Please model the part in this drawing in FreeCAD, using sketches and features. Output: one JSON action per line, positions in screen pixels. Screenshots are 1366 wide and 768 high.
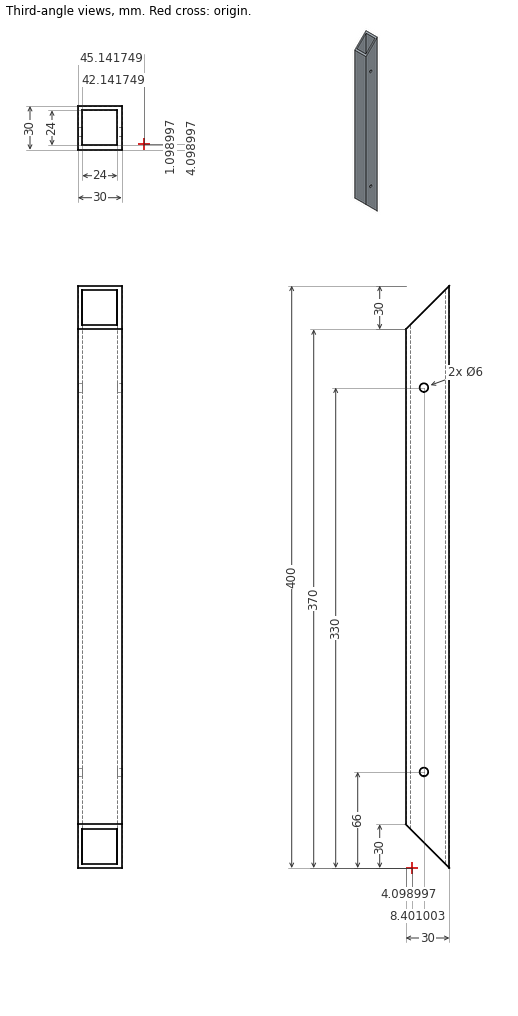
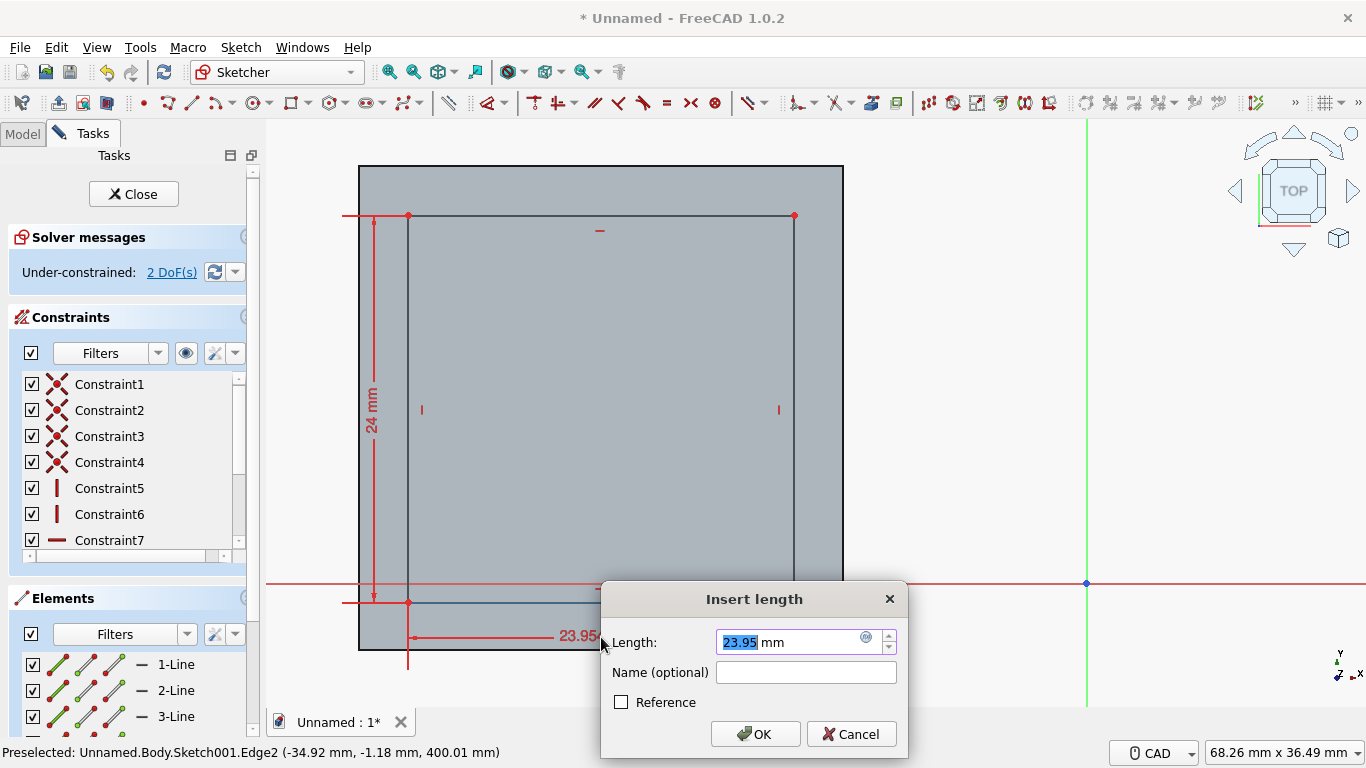
{"action": "type", "text": "24"}
{"action": "key", "text": "Return"}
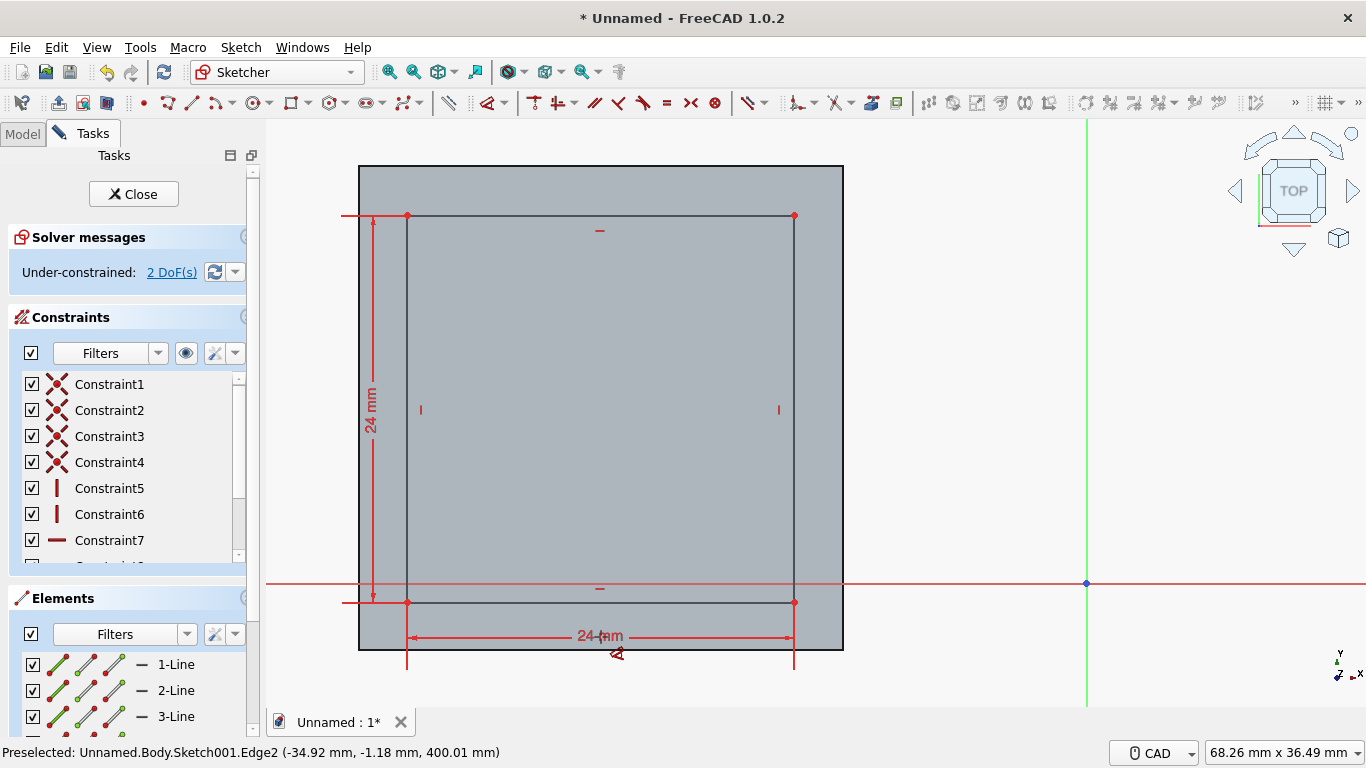
{"action": "scroll", "coordinate": [407, 603], "scroll_direction": "up", "scroll_amount": 5}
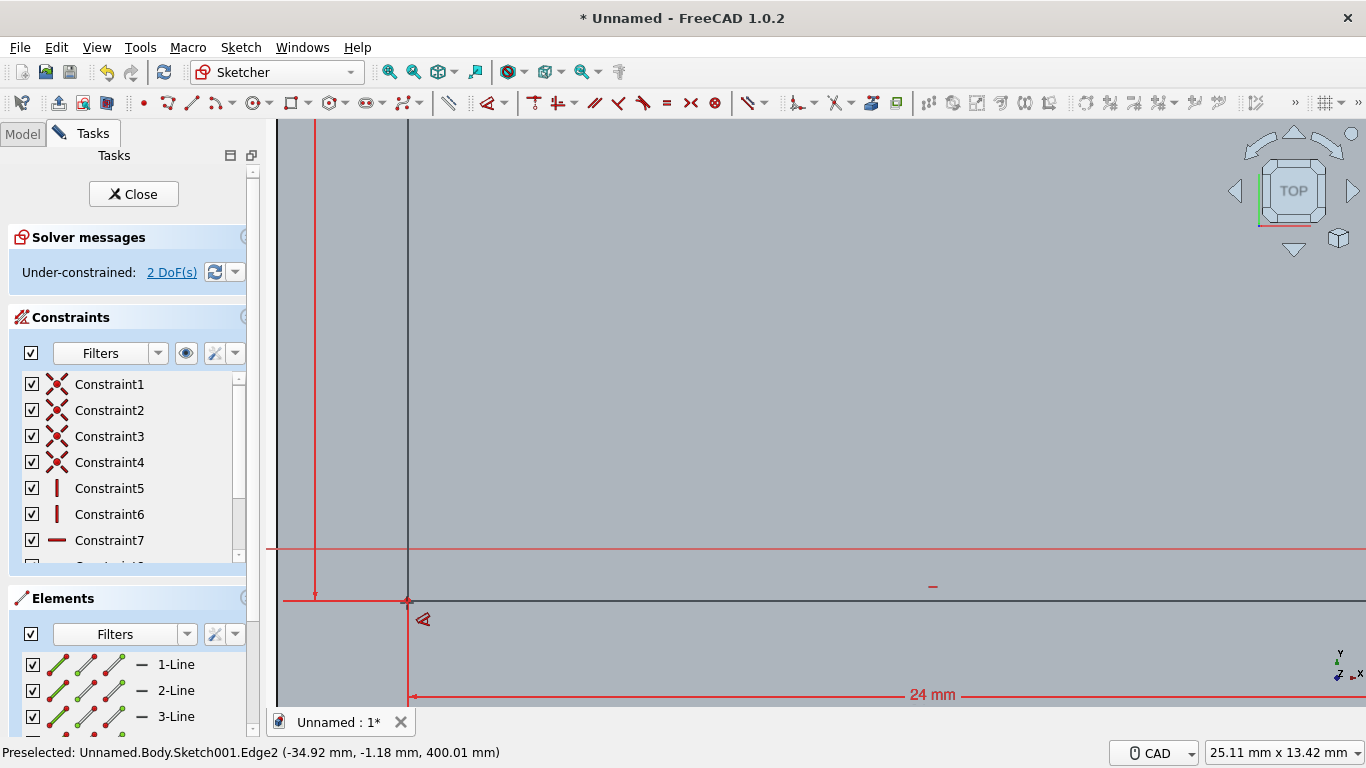
{"action": "left_click", "coordinate": [408, 601]}
{"action": "left_click", "coordinate": [374, 575]}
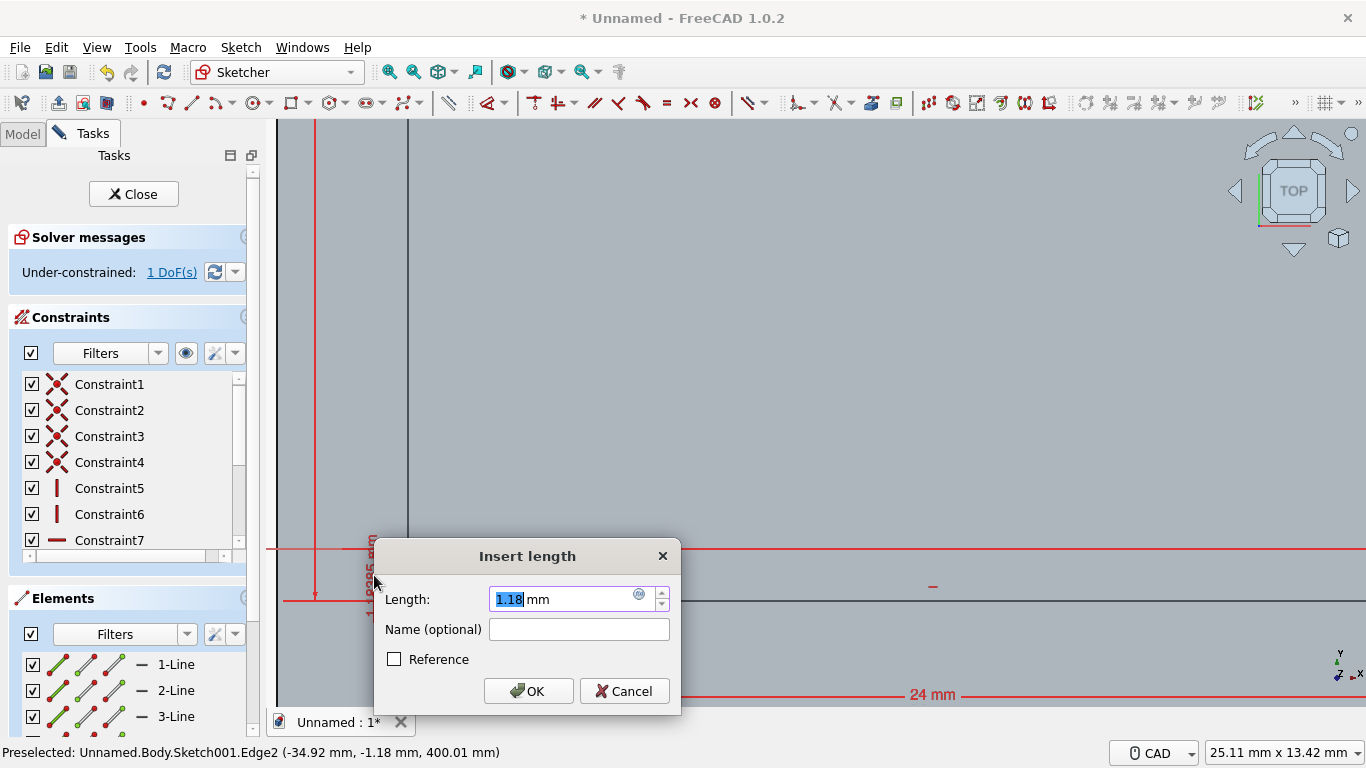
{"action": "type", "text": "1.098997"}
{"action": "key", "text": "Return"}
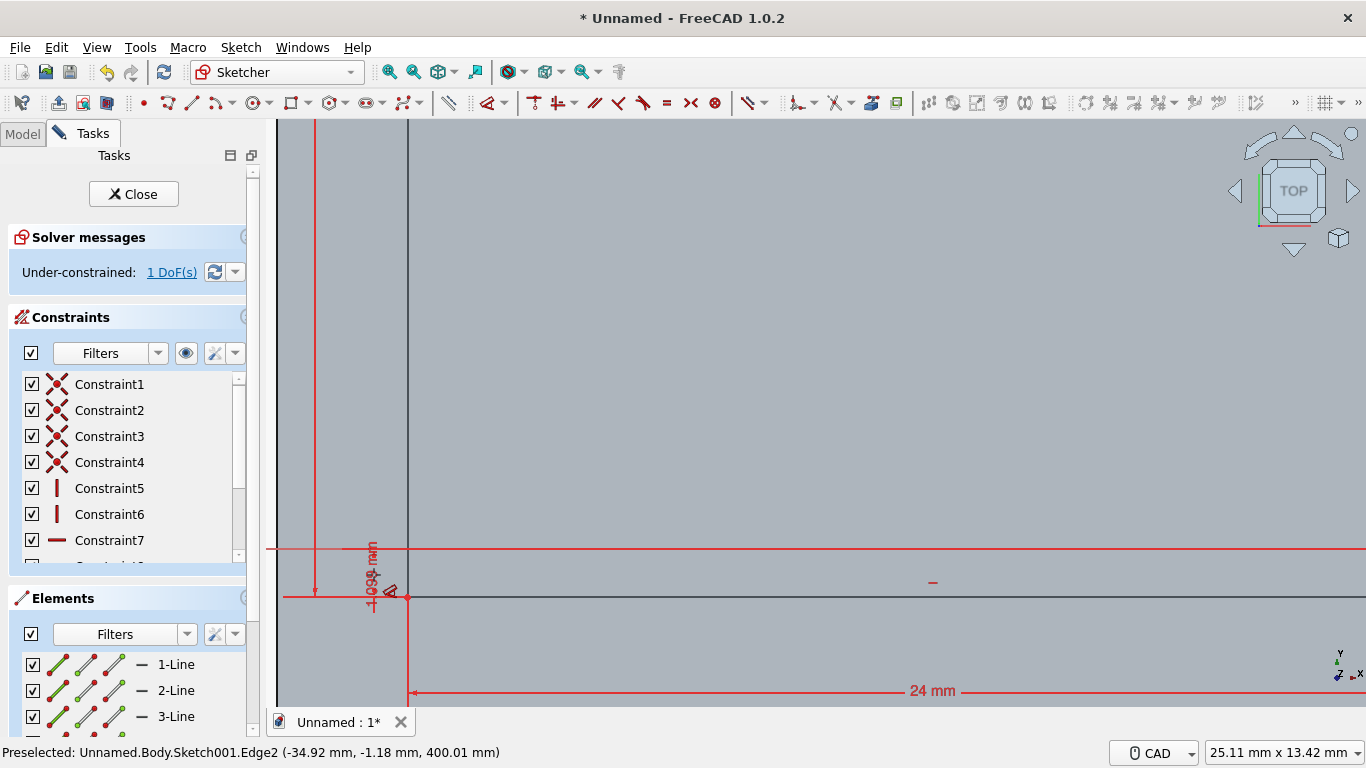
{"action": "scroll", "coordinate": [408, 612], "scroll_direction": "down", "scroll_amount": 5}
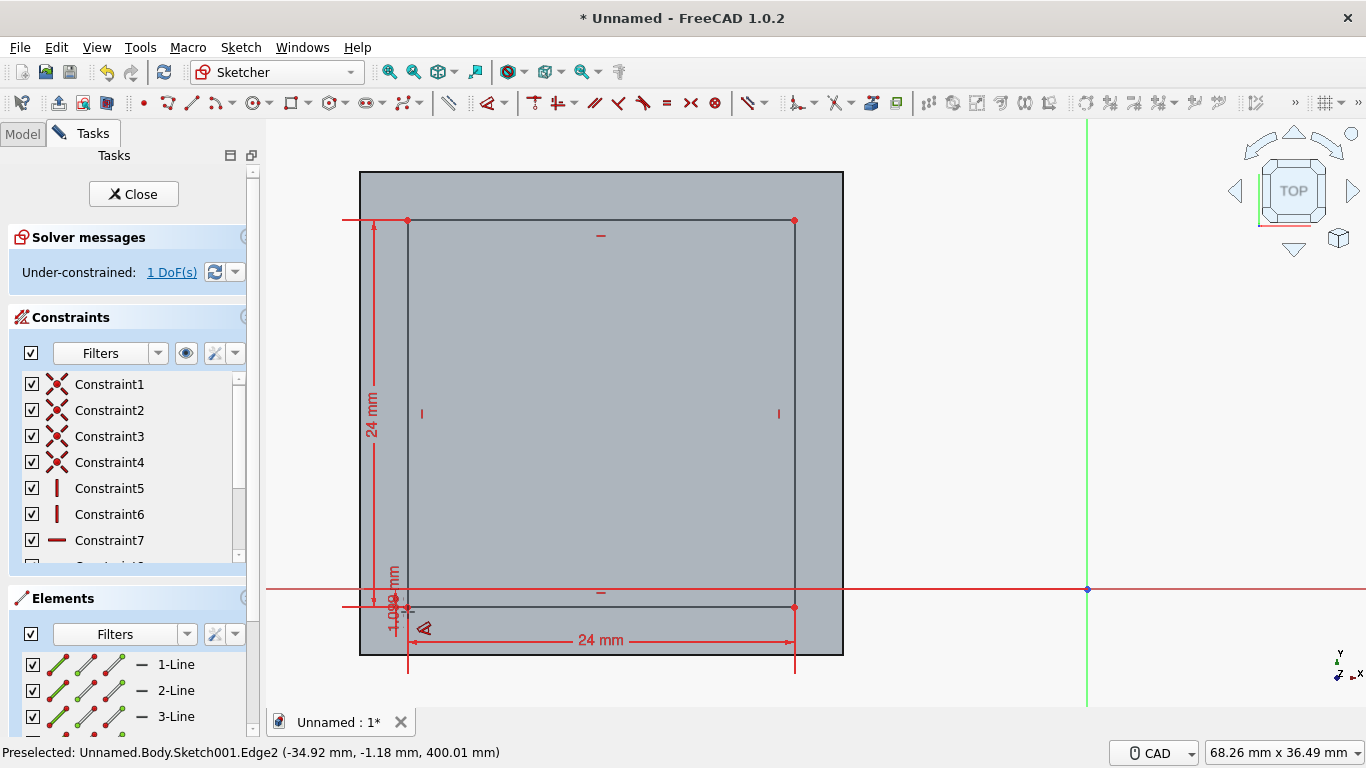
{"action": "left_click", "coordinate": [408, 220]}
{"action": "left_click", "coordinate": [748, 186]}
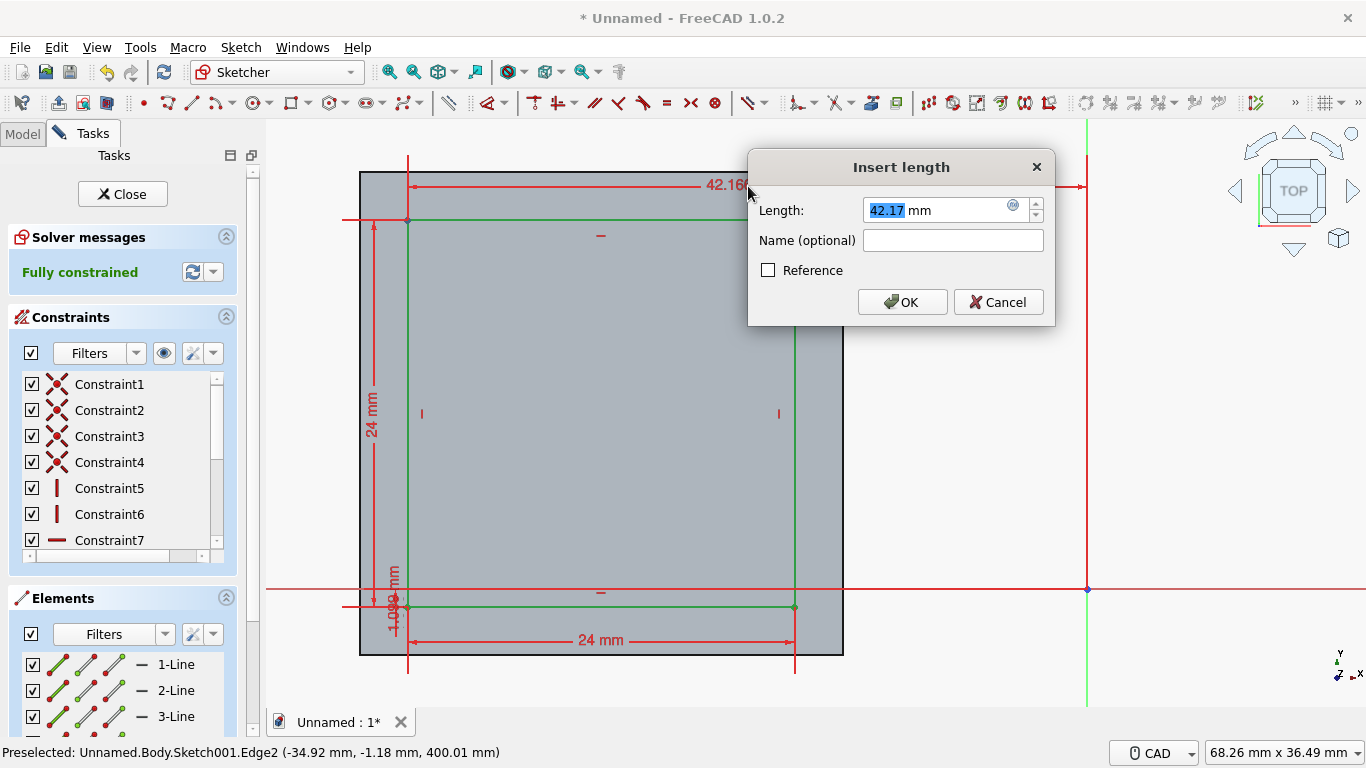
{"action": "type", "text": "42.141749"}
{"action": "key", "text": "Return"}
{"action": "key", "text": "Escape"}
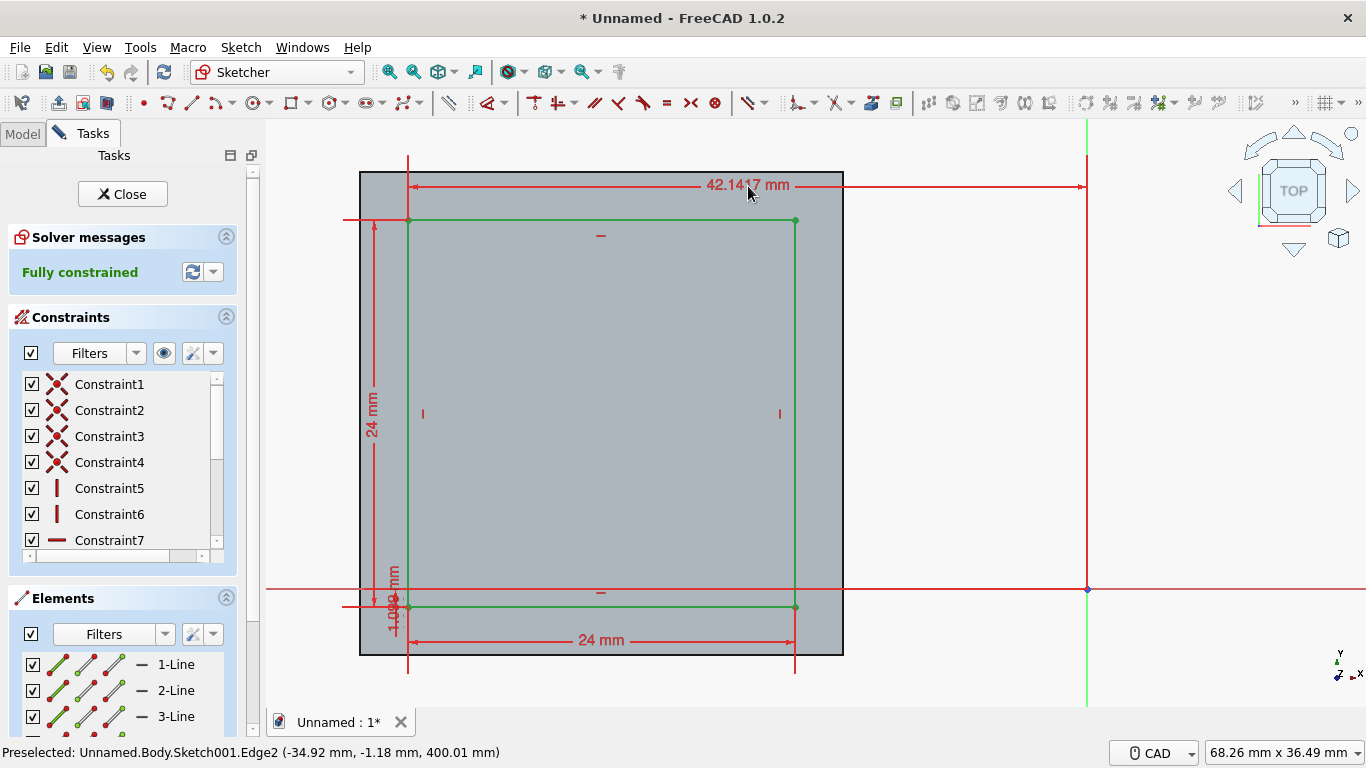
{"action": "left_click", "coordinate": [123, 194]}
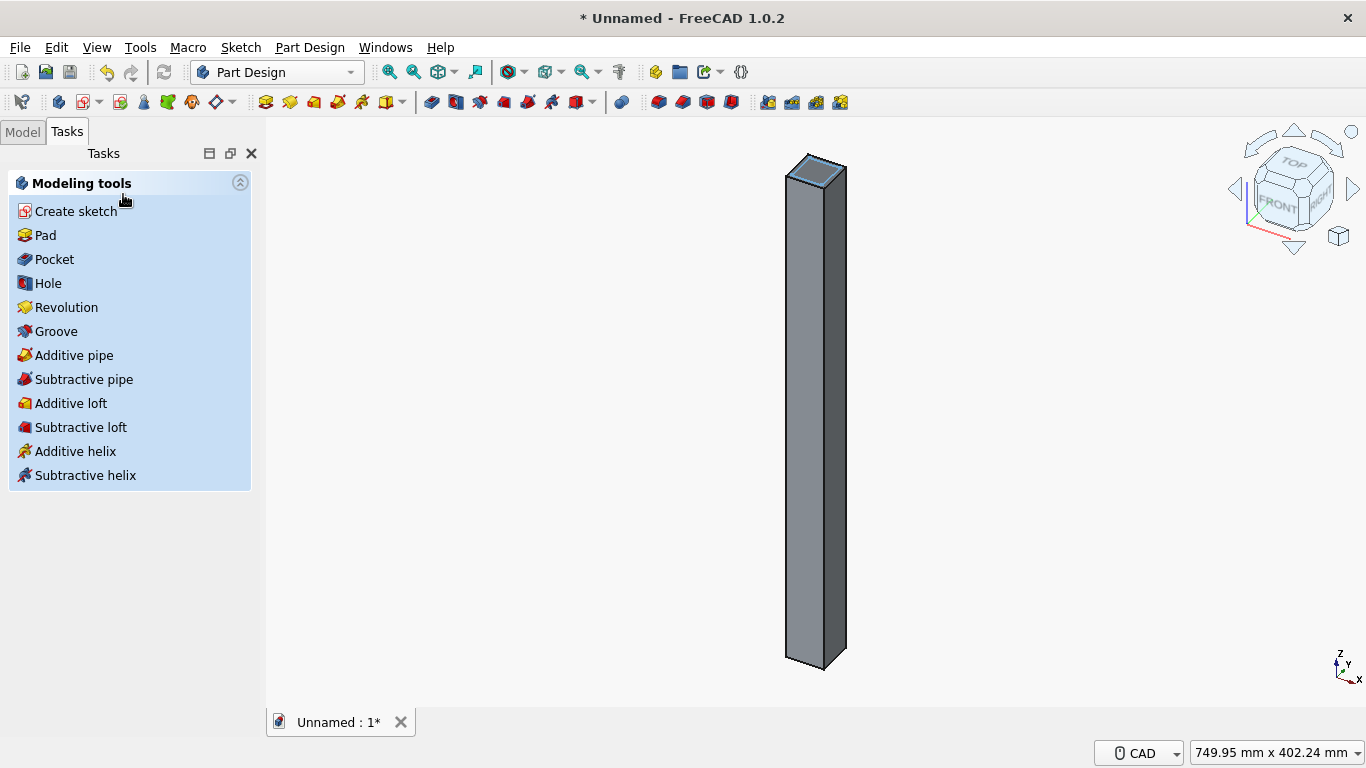
{"action": "left_click", "coordinate": [432, 102]}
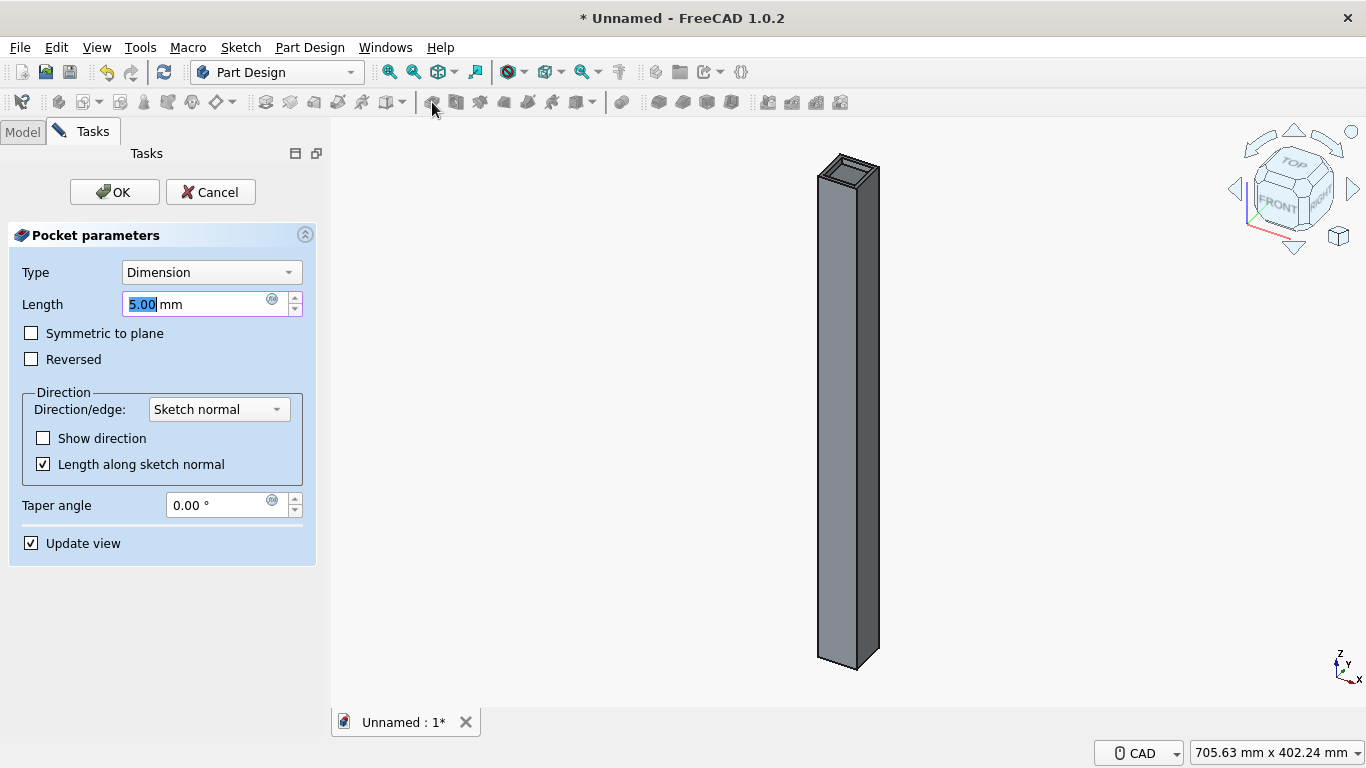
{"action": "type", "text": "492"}
{"action": "key", "text": "Tab"}